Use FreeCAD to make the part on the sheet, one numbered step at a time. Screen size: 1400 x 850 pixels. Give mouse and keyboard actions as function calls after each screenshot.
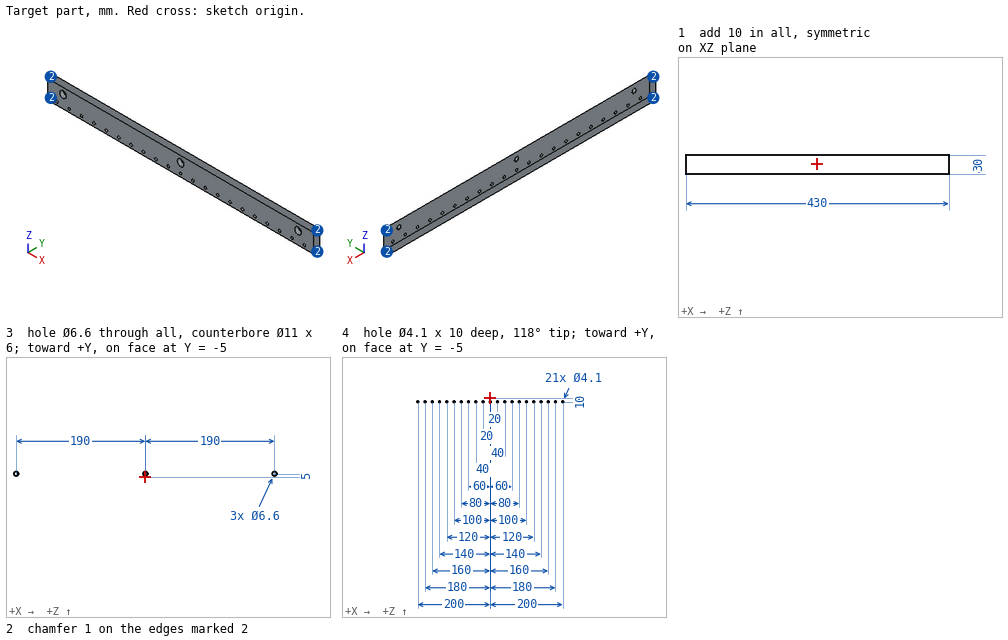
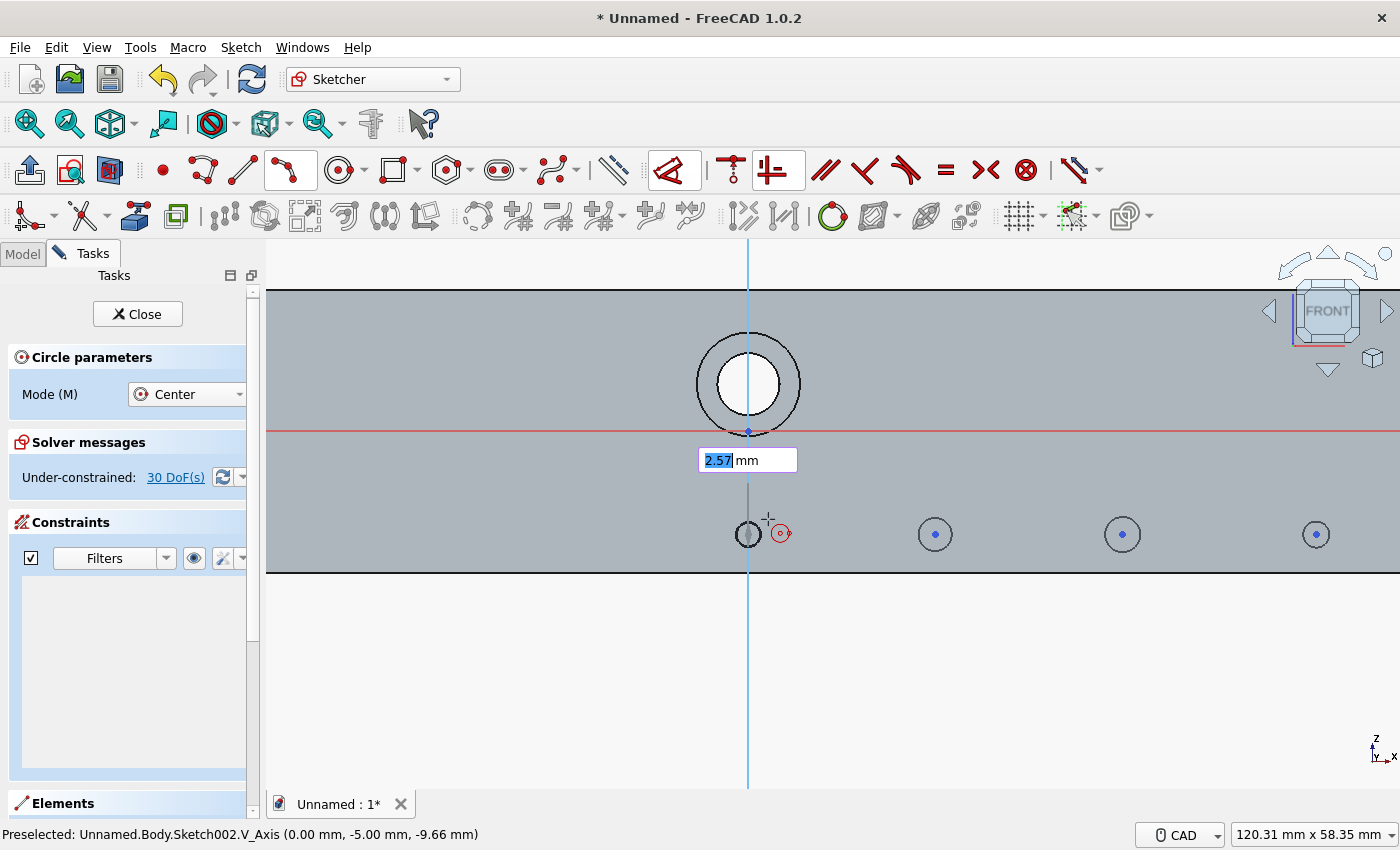
click(767, 519)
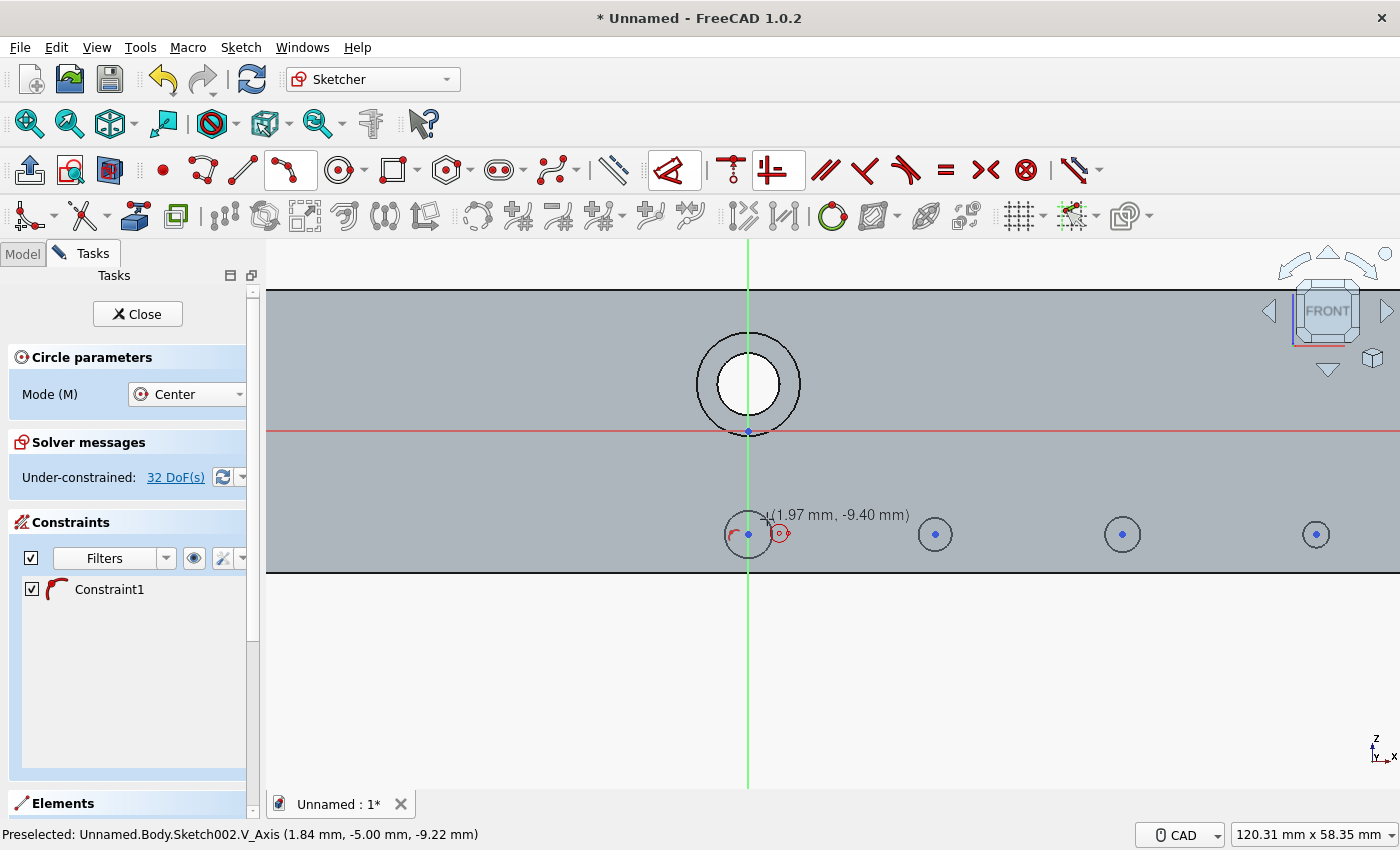
scroll(768, 519, down, 9)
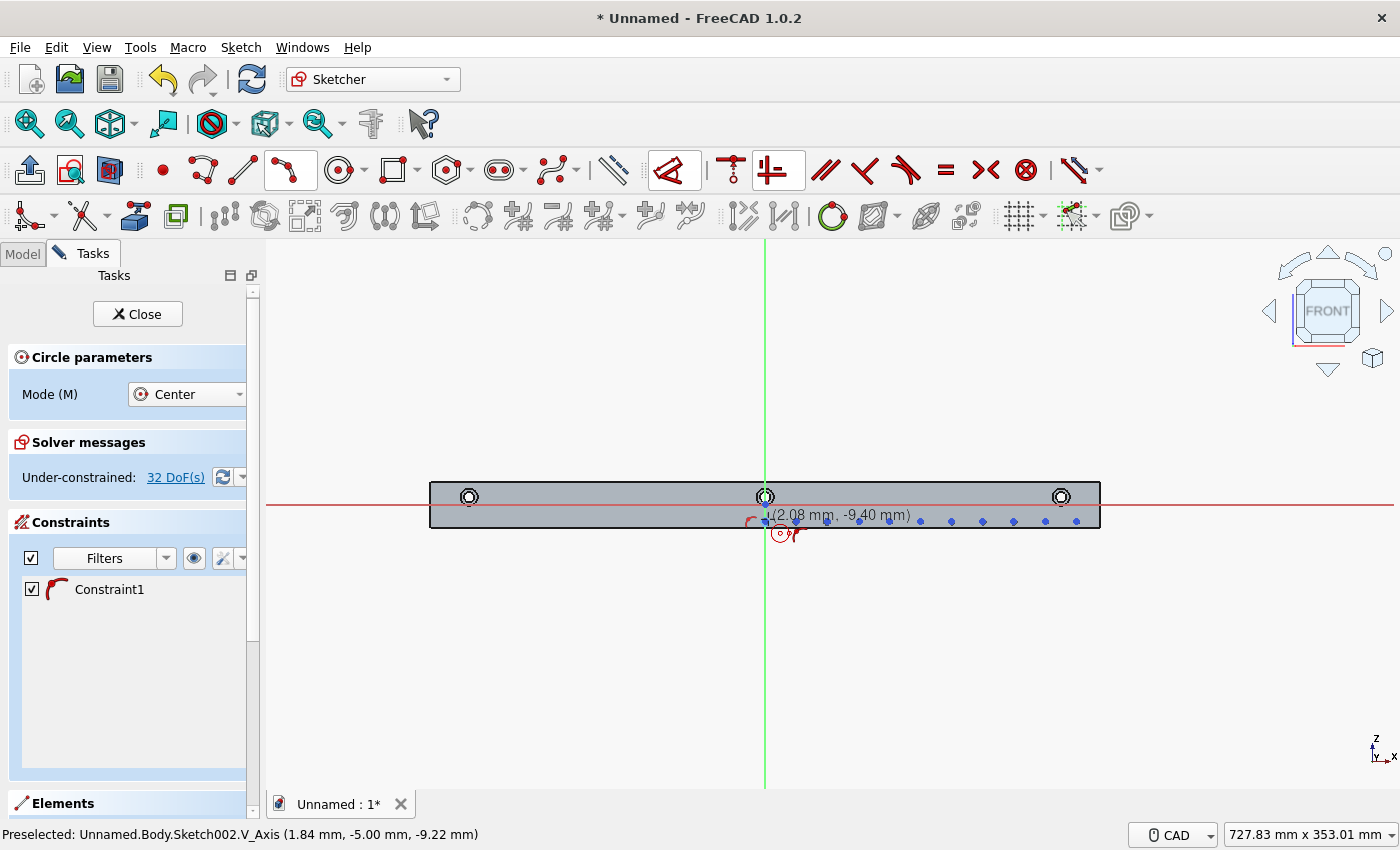
click(734, 521)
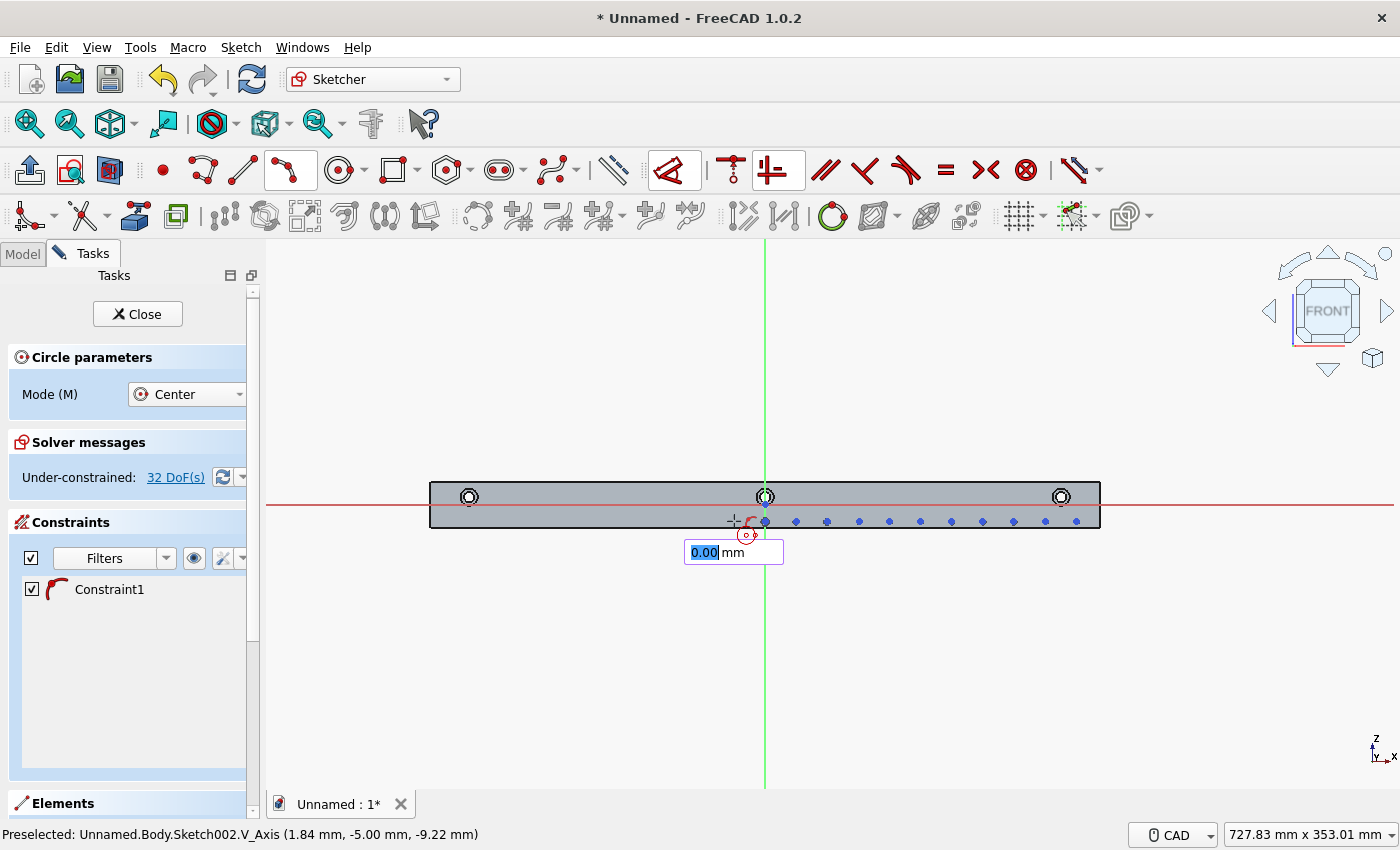
scroll(736, 523, up, 9)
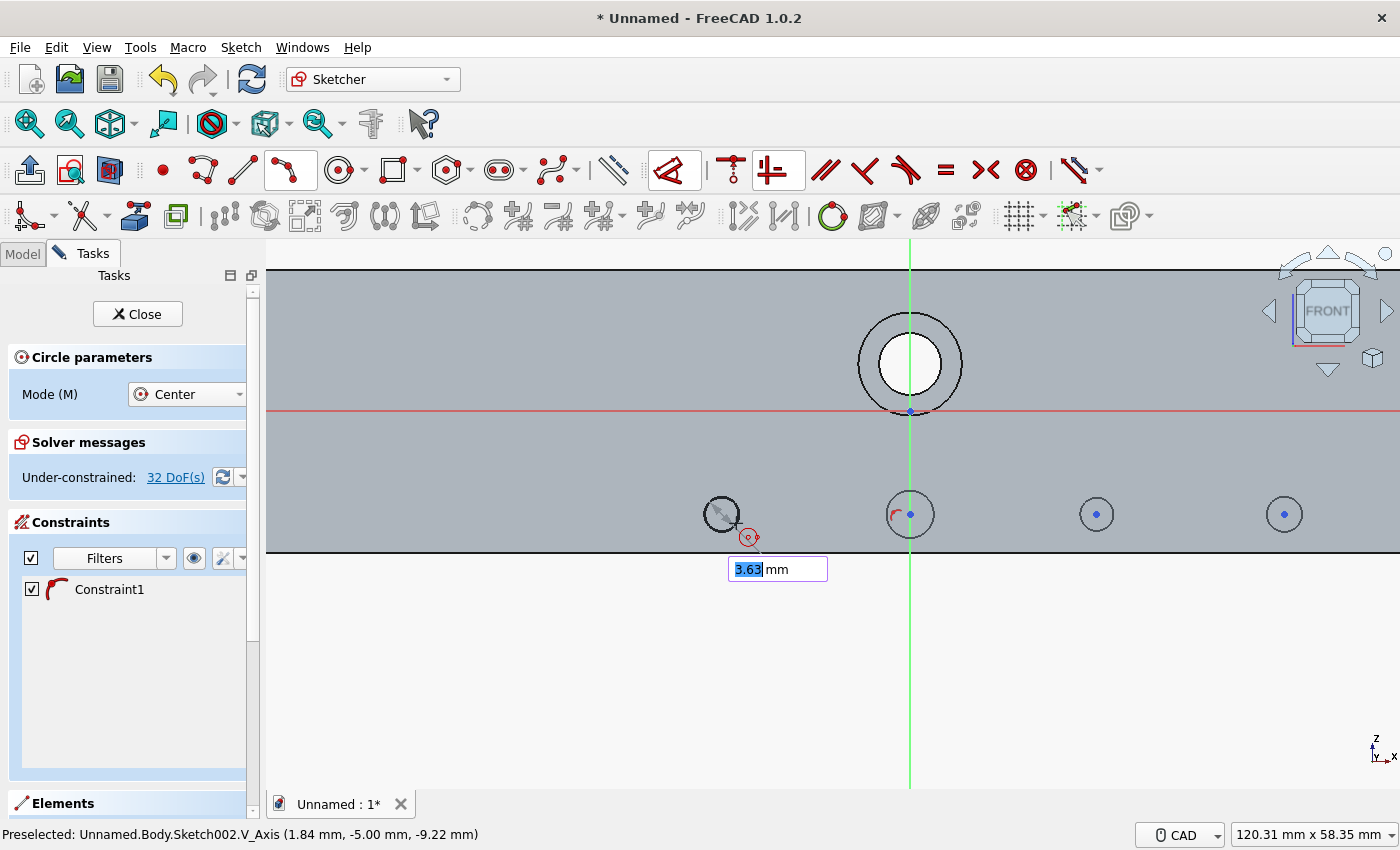
click(735, 519)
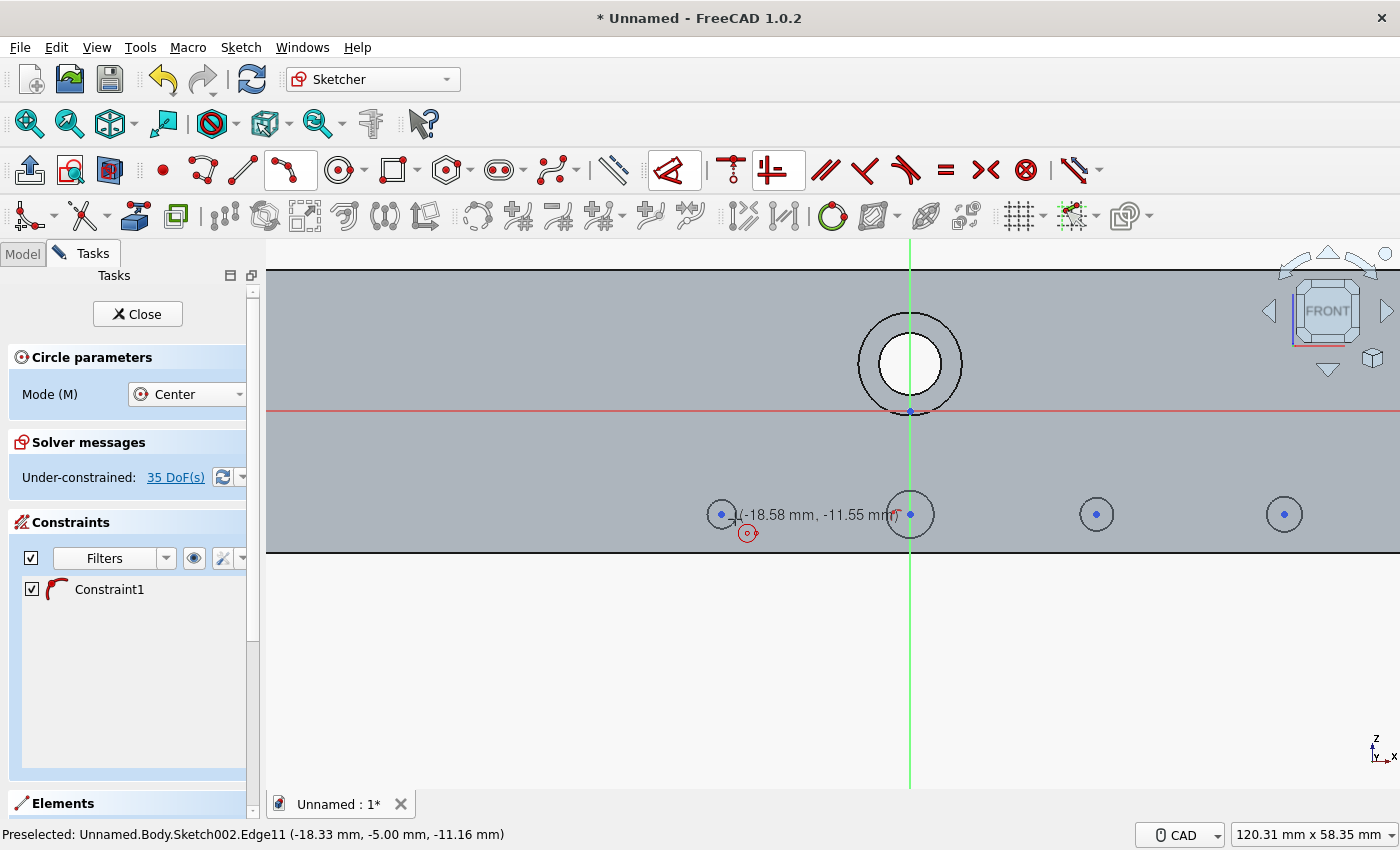
scroll(736, 523, down, 9)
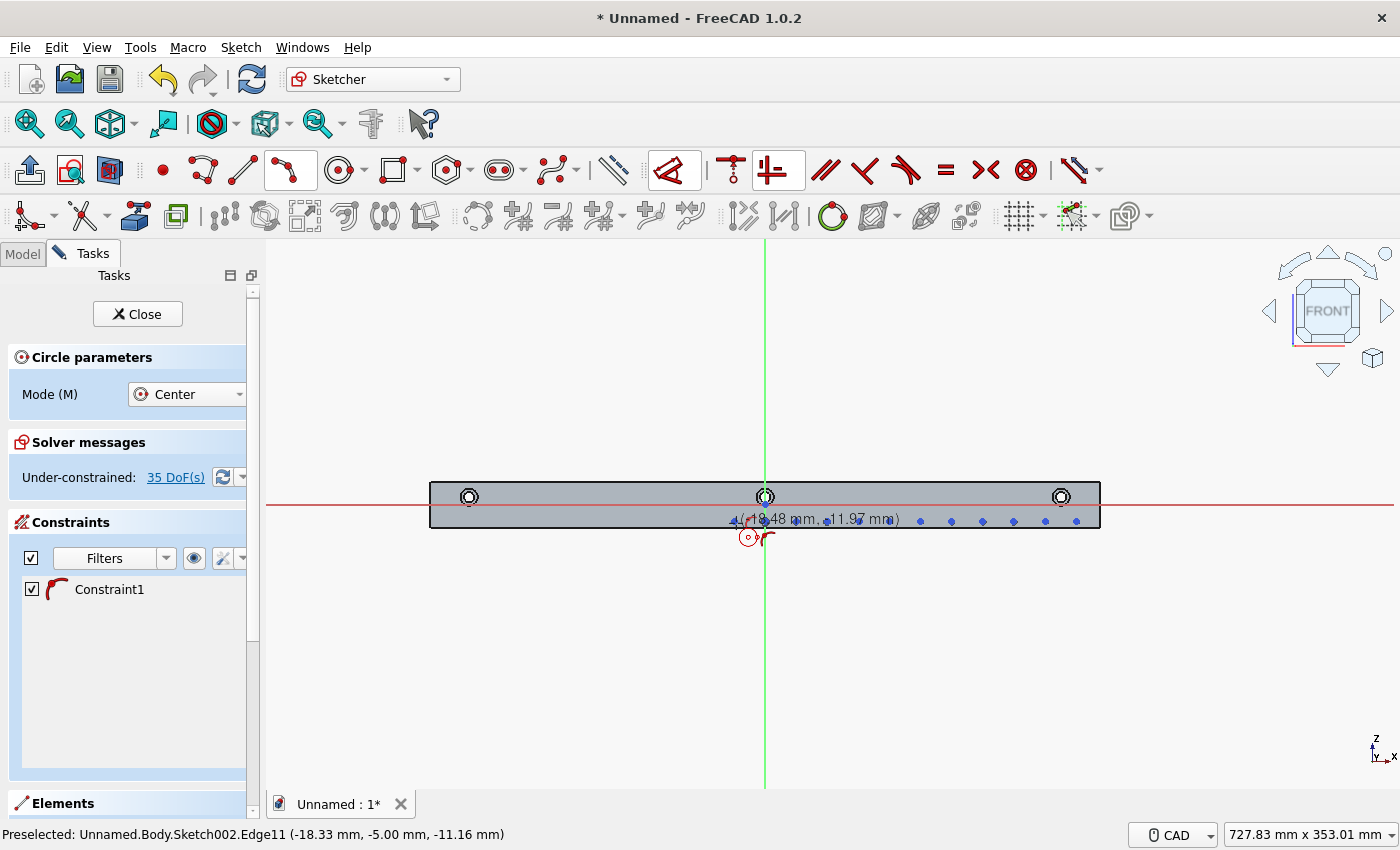
click(703, 521)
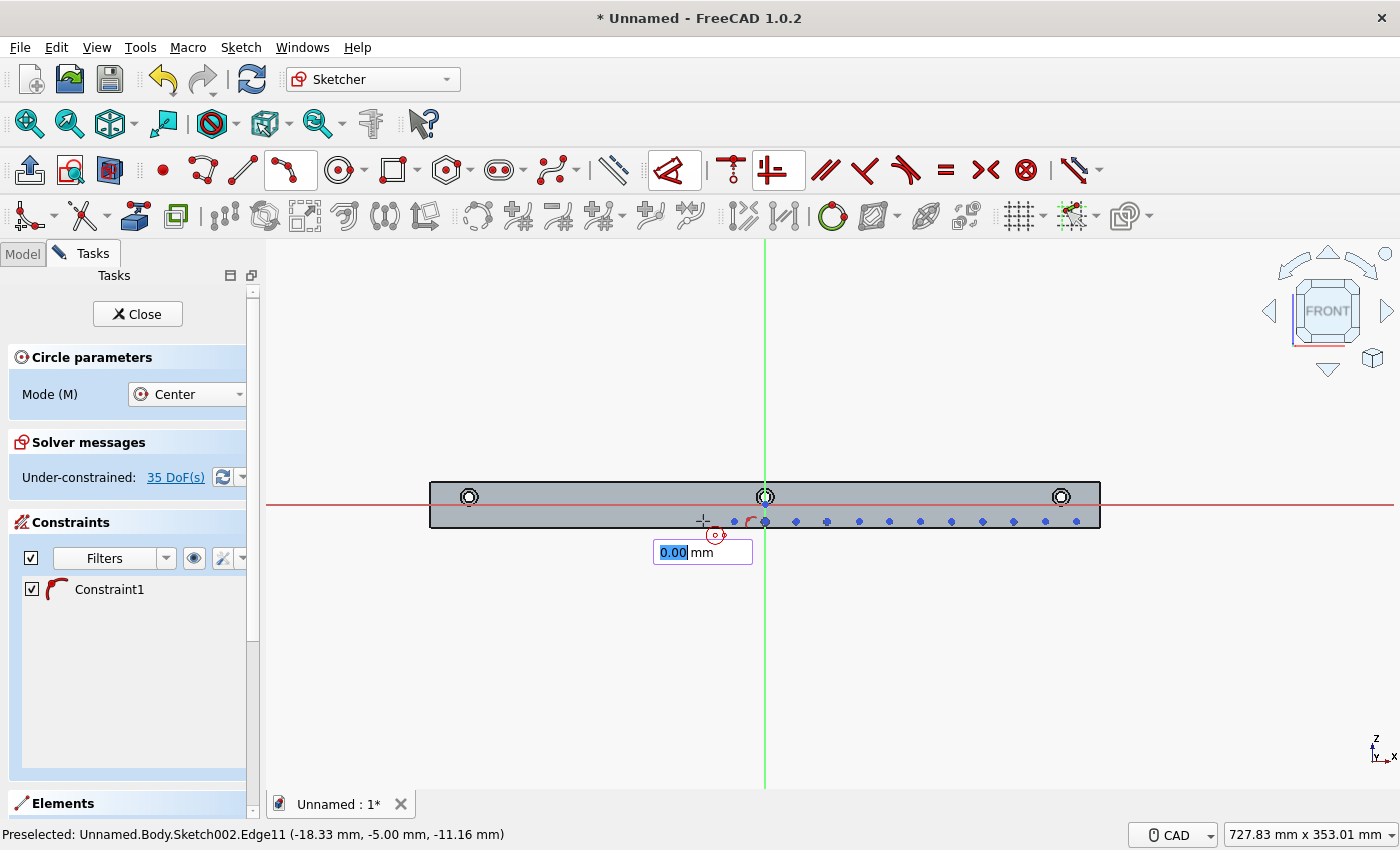
scroll(705, 523, up, 9)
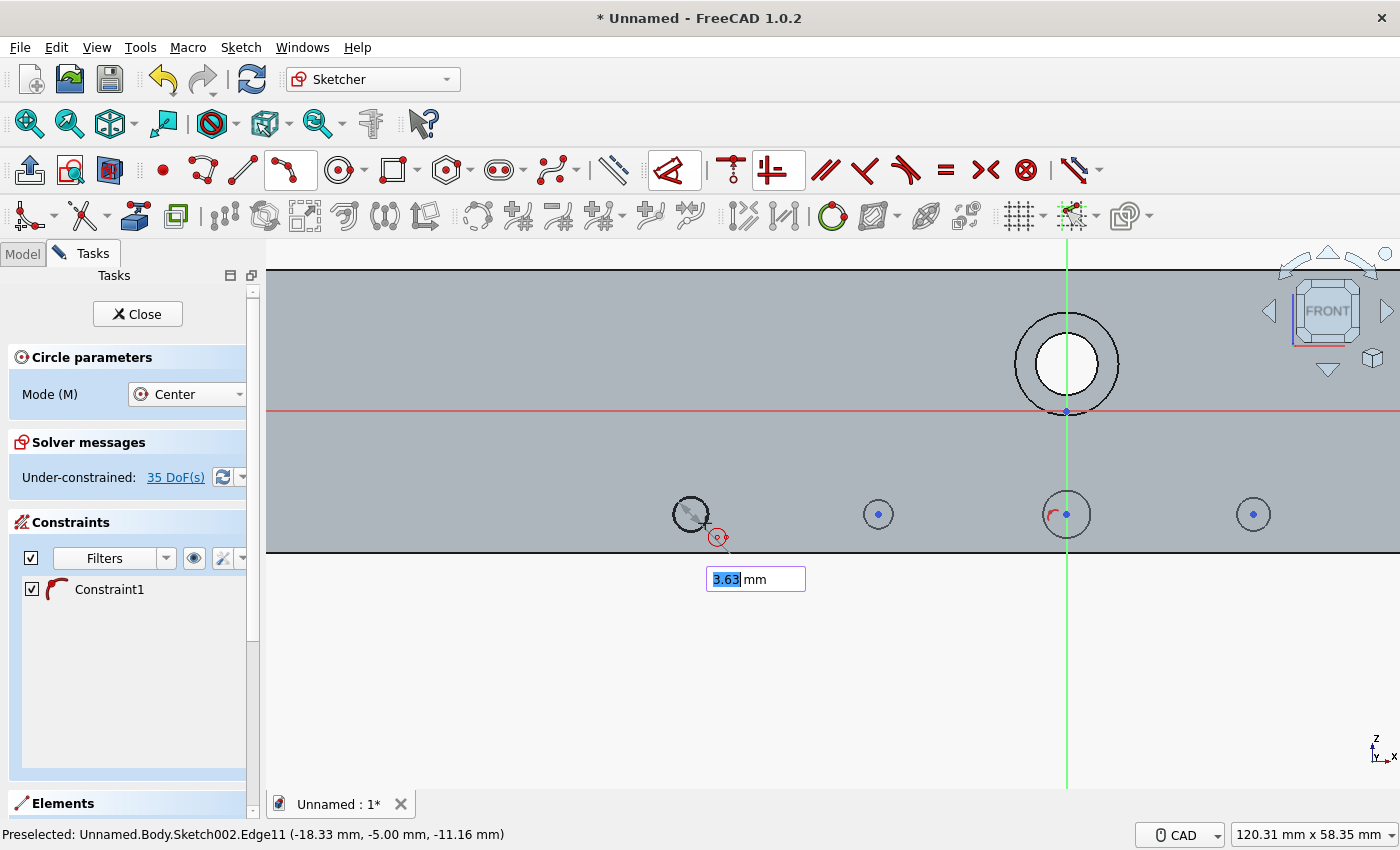
click(703, 519)